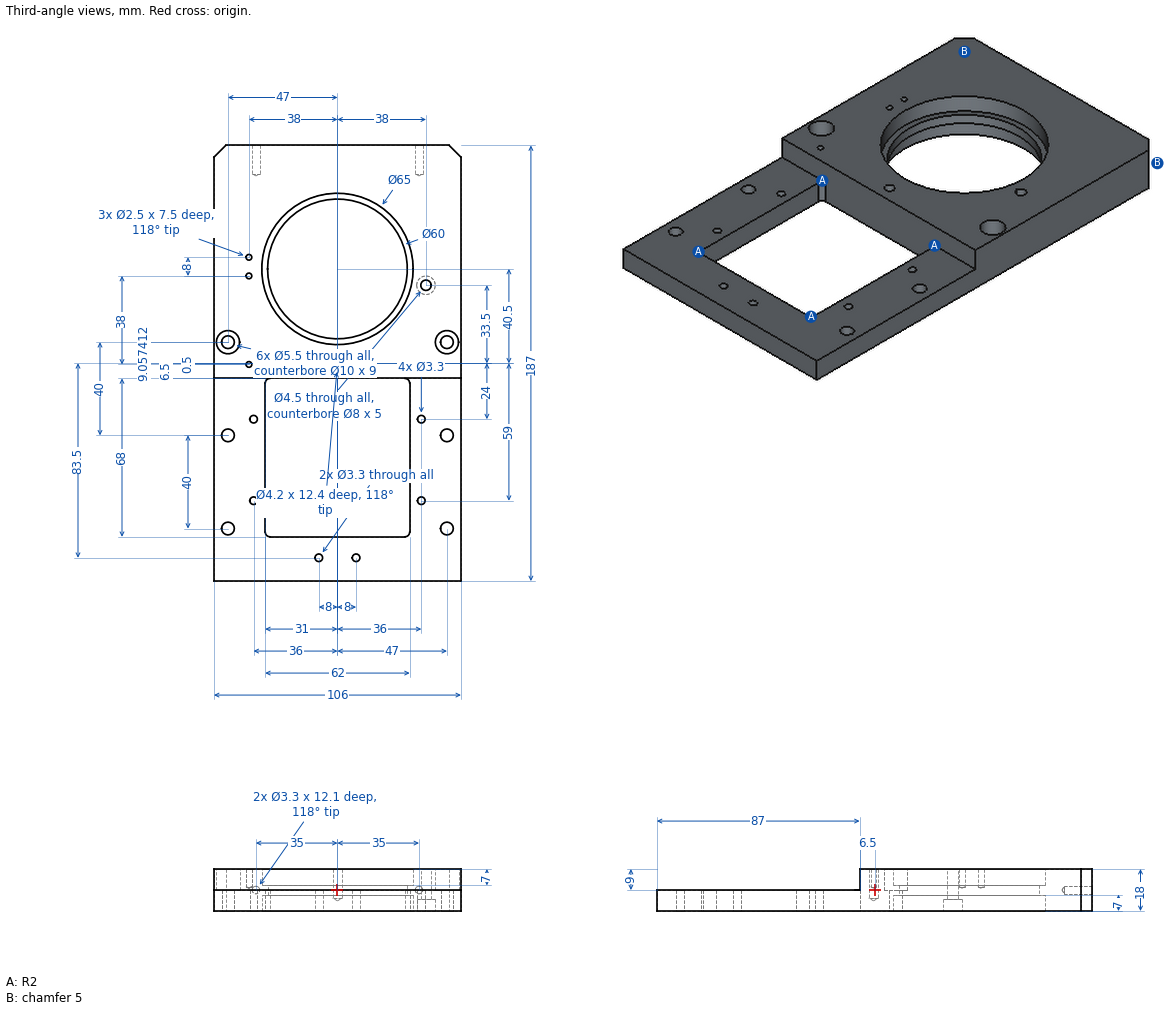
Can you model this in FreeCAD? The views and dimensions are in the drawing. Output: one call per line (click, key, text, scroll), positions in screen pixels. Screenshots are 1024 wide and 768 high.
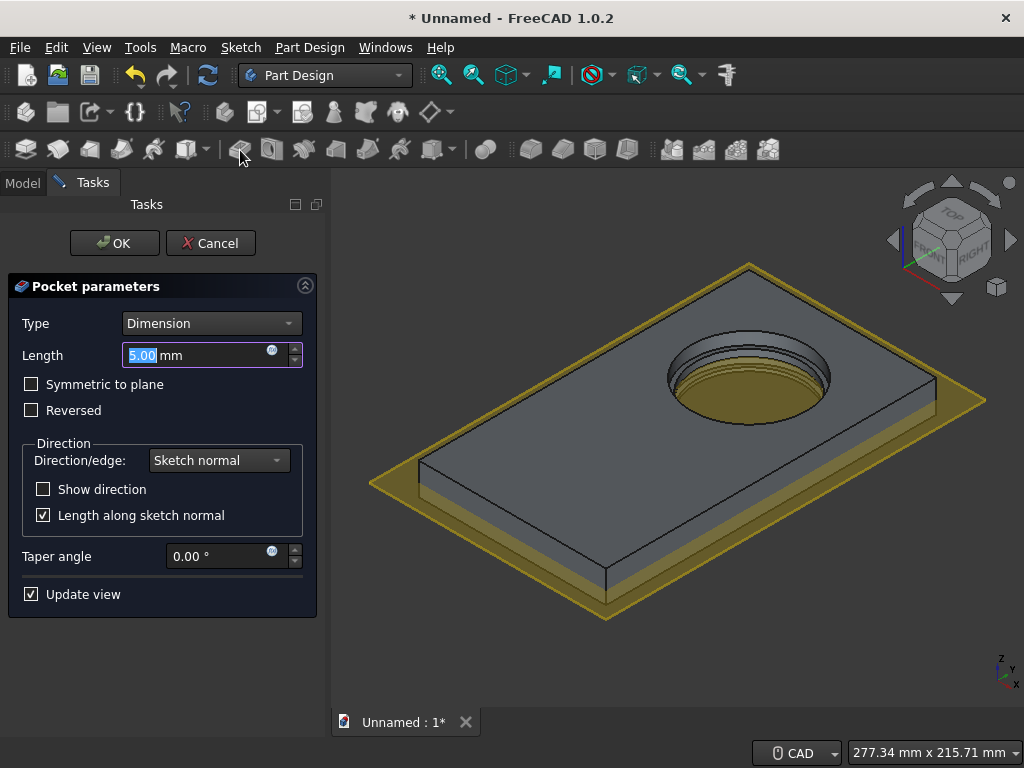
text(7)
key(Tab)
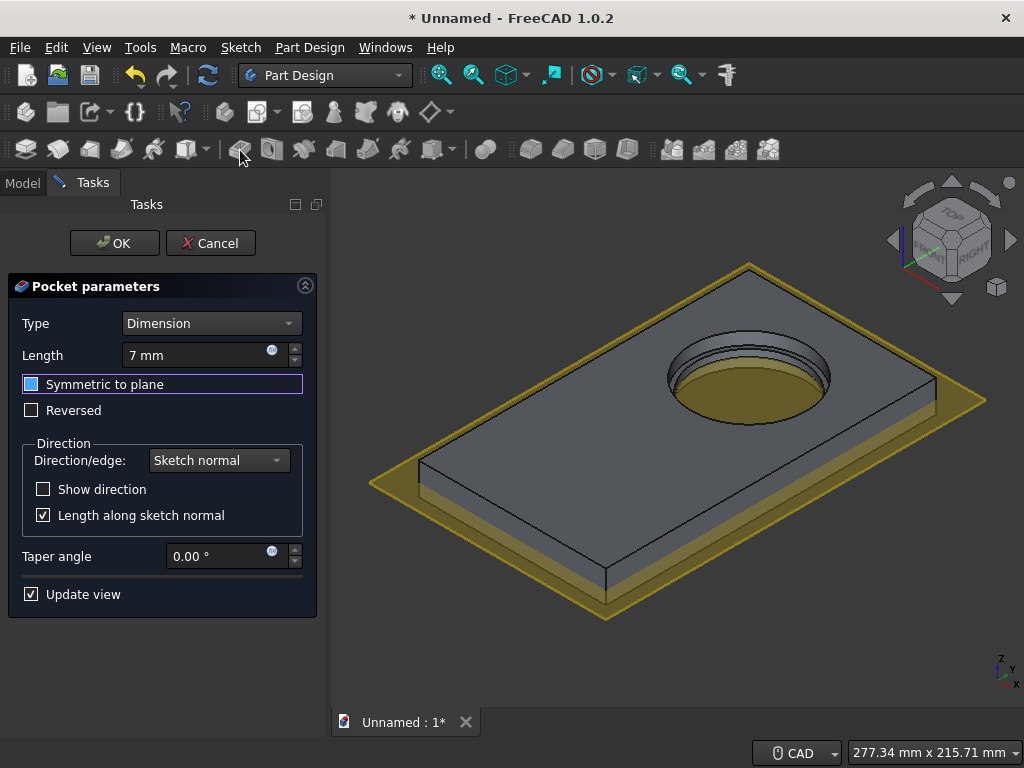
click(115, 243)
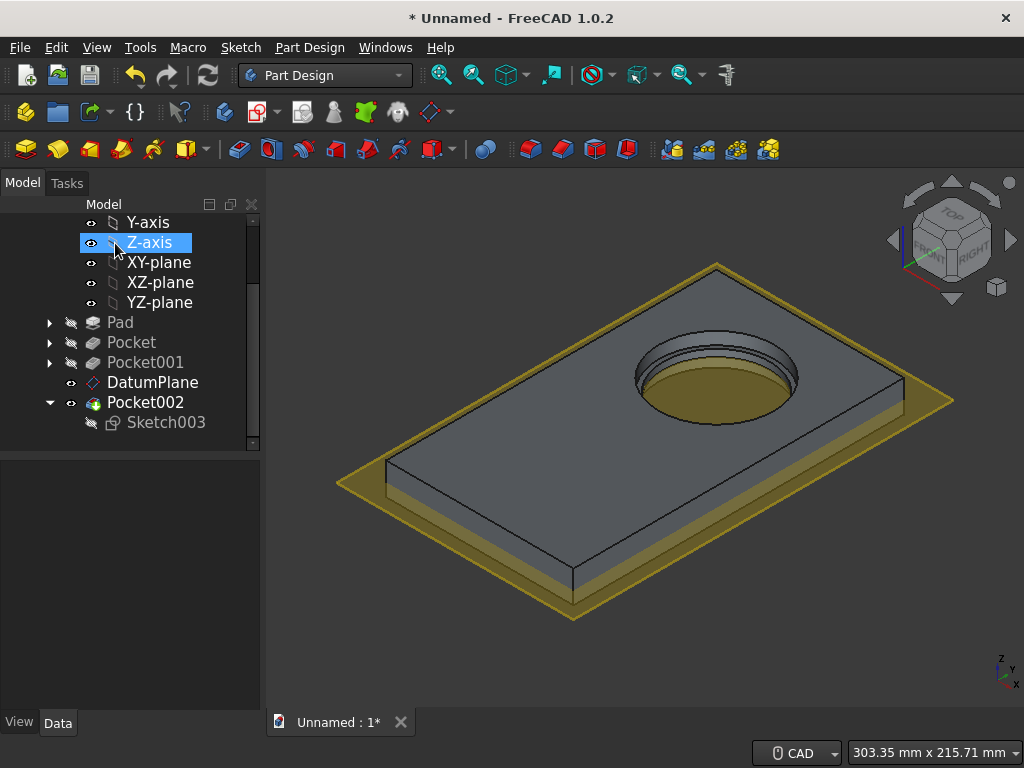
click(116, 383)
key(space)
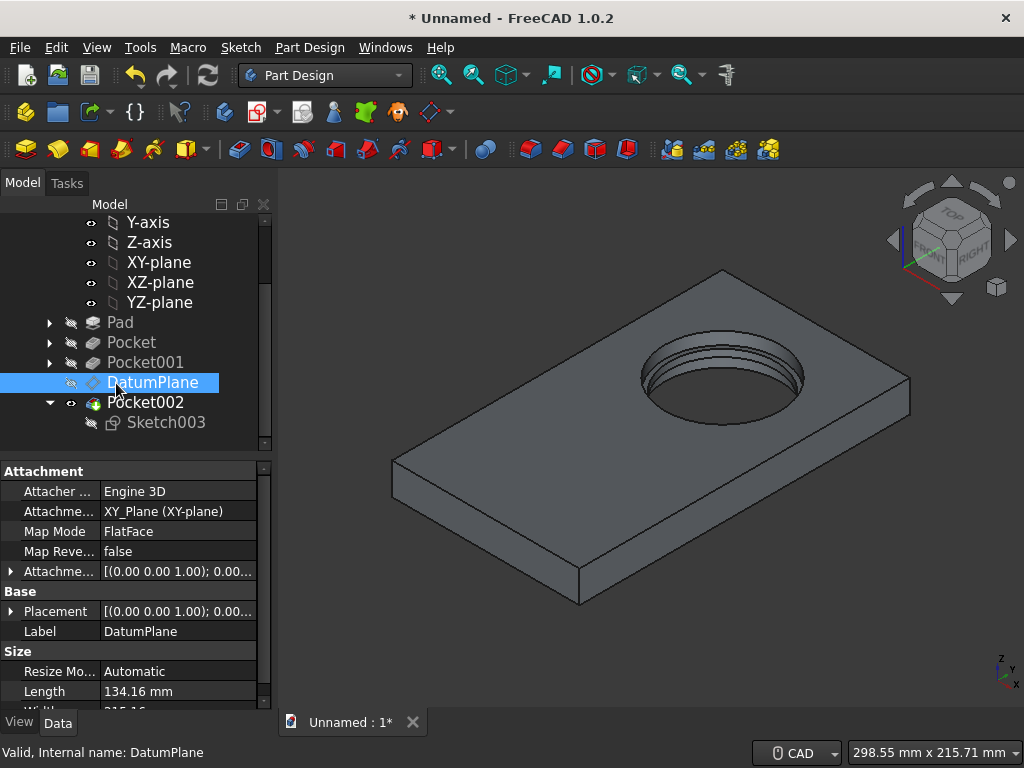
click(557, 473)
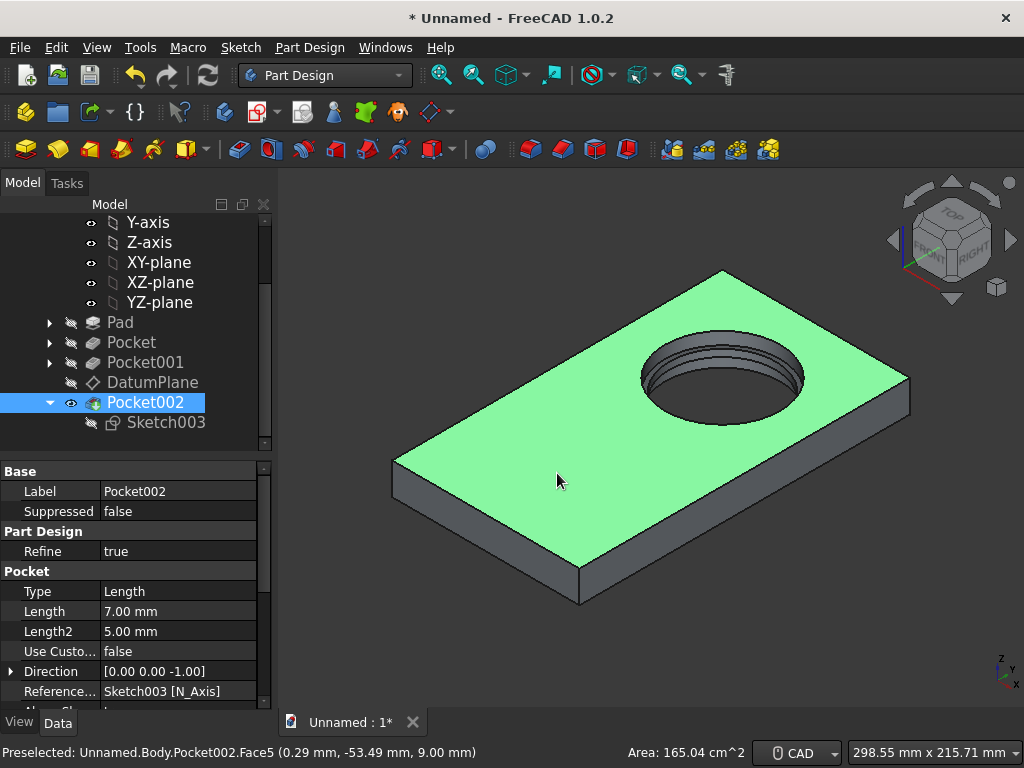
click(258, 112)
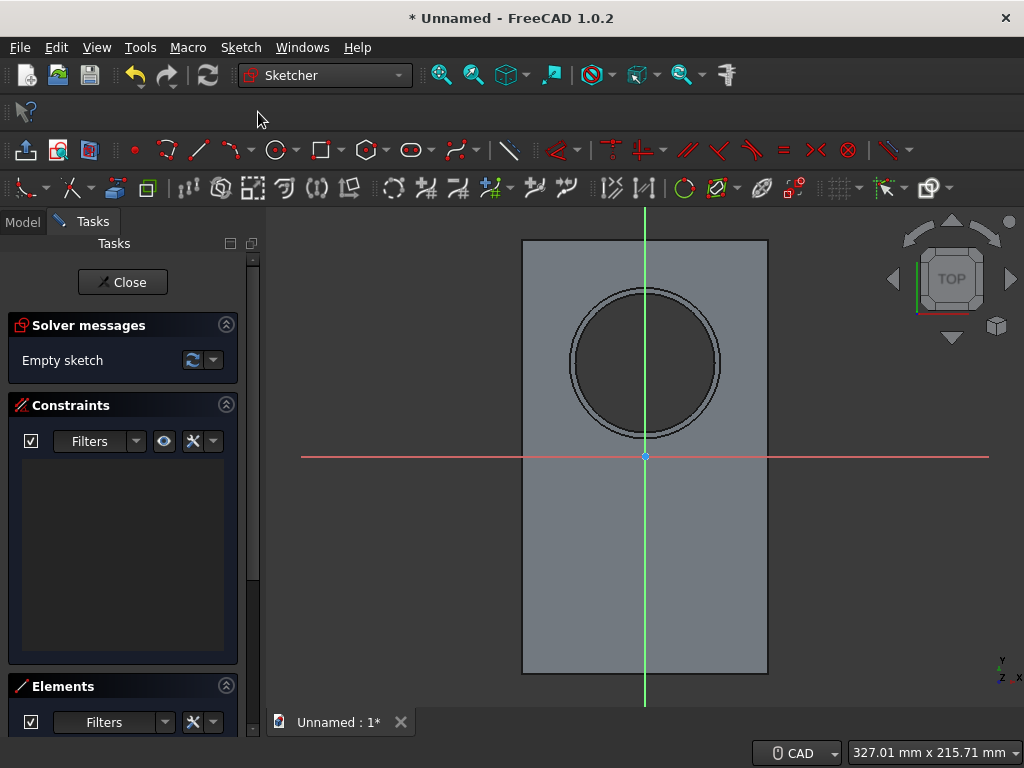
scroll(728, 648, up, 3)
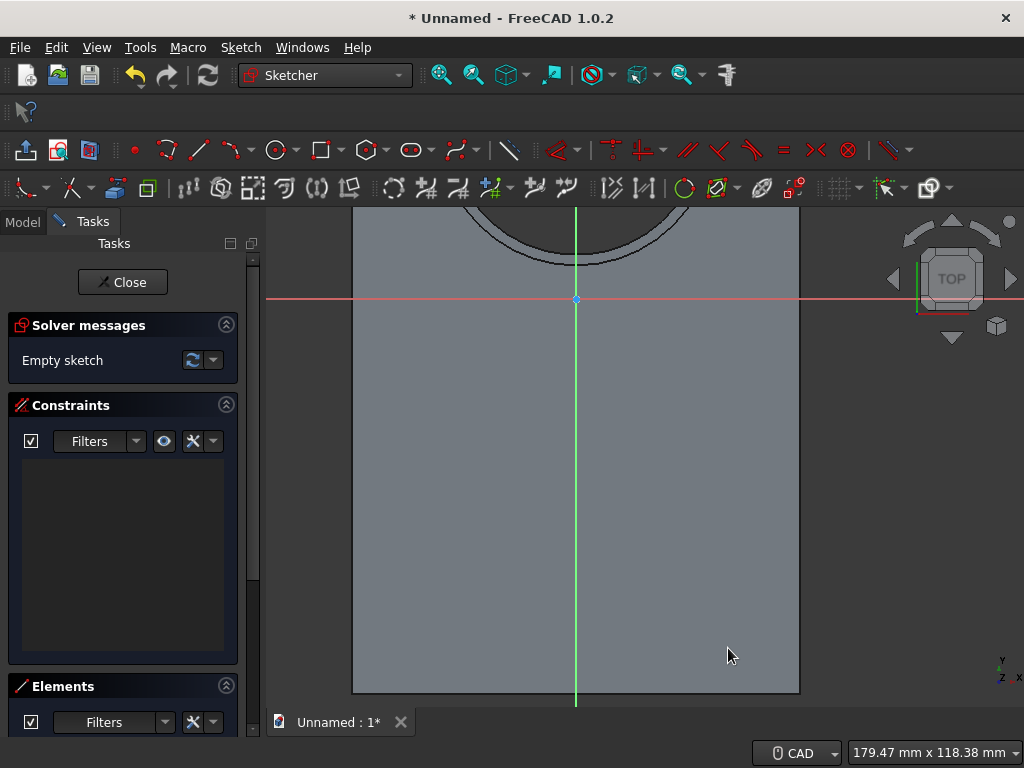
click(322, 150)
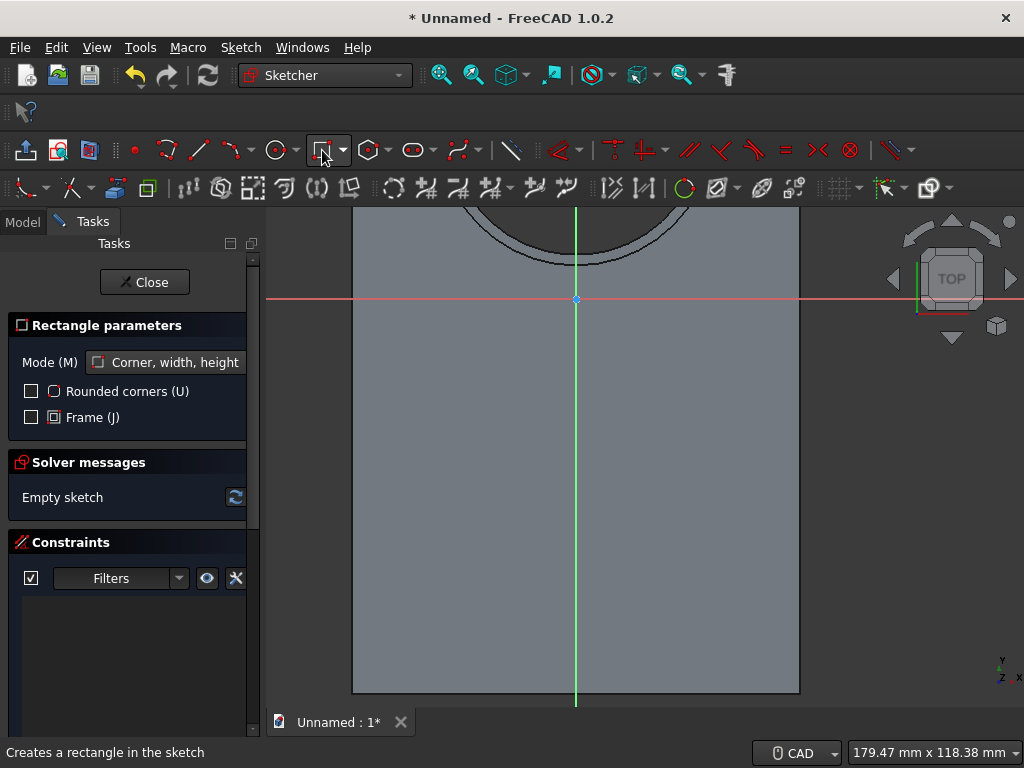
click(445, 327)
click(707, 614)
key(Escape)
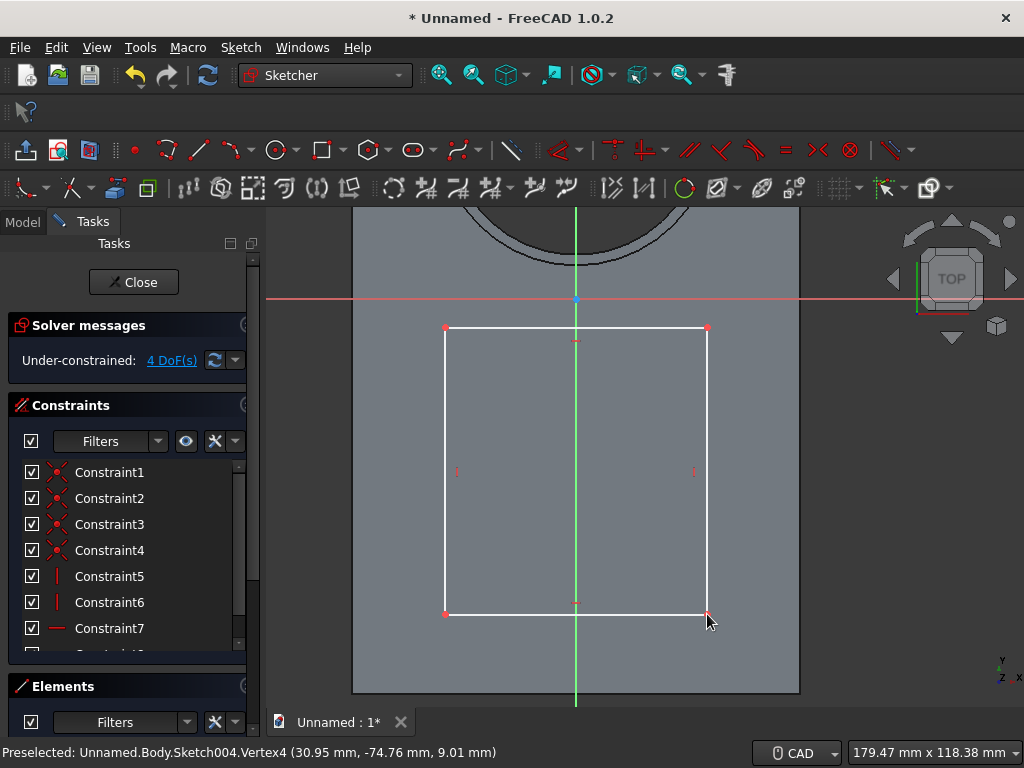
click(558, 150)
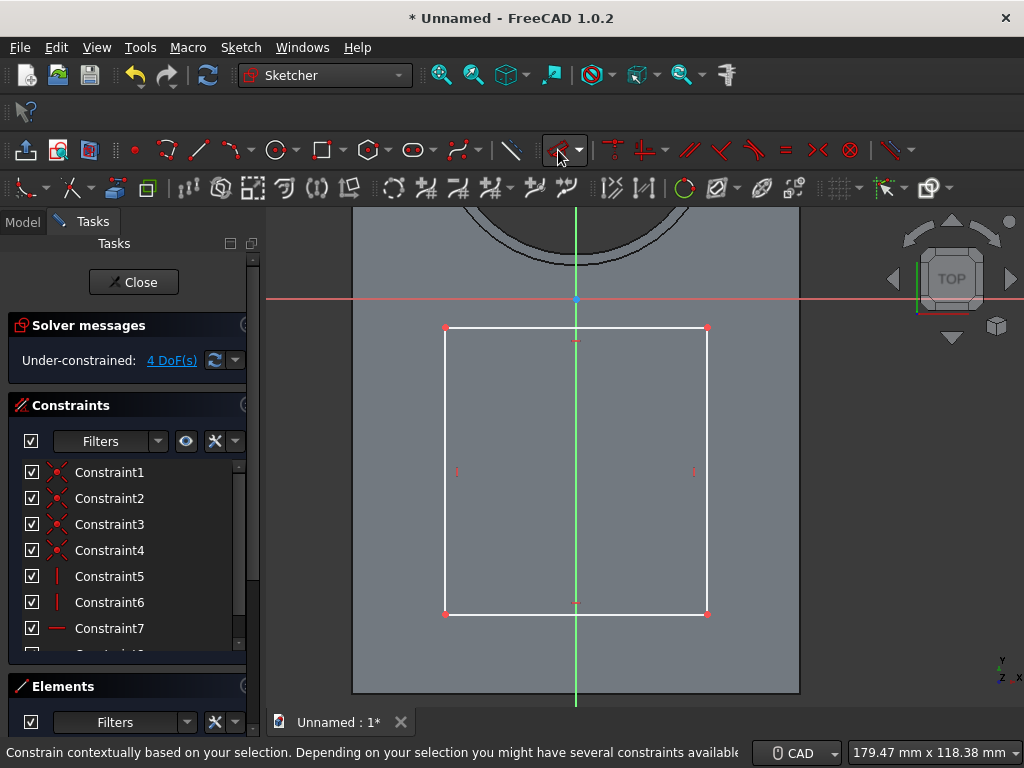
click(445, 414)
click(411, 471)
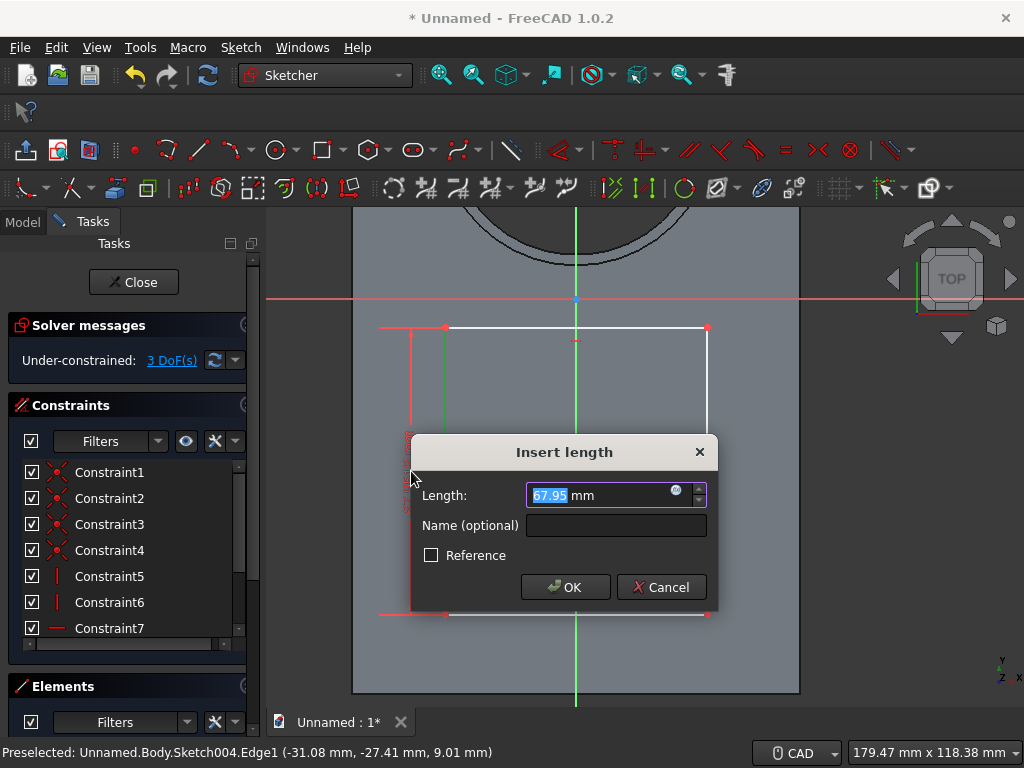
text(68)
key(Return)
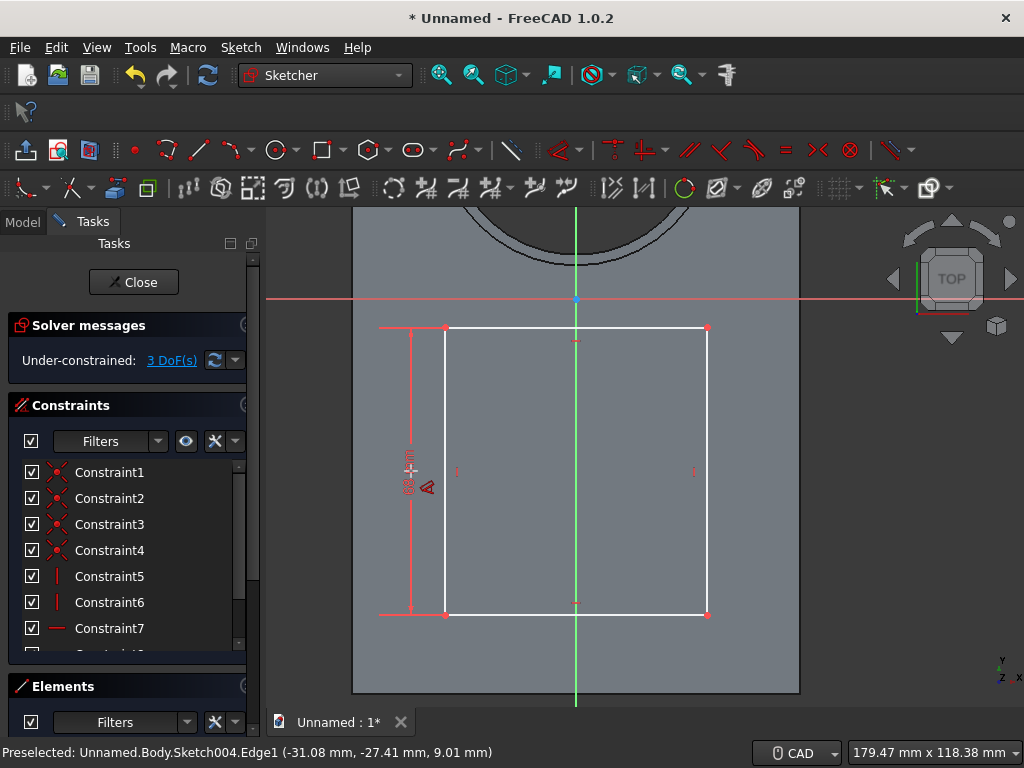
click(524, 615)
click(516, 649)